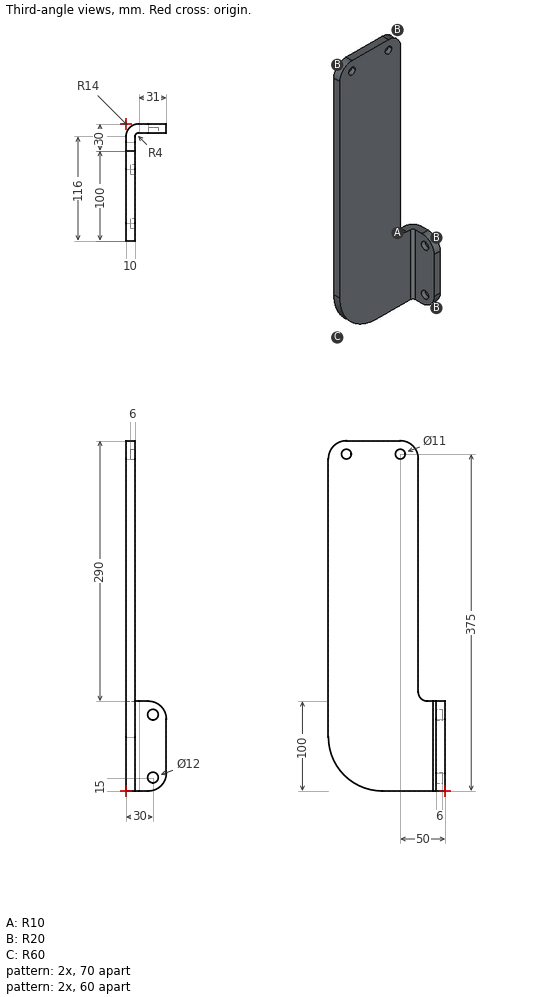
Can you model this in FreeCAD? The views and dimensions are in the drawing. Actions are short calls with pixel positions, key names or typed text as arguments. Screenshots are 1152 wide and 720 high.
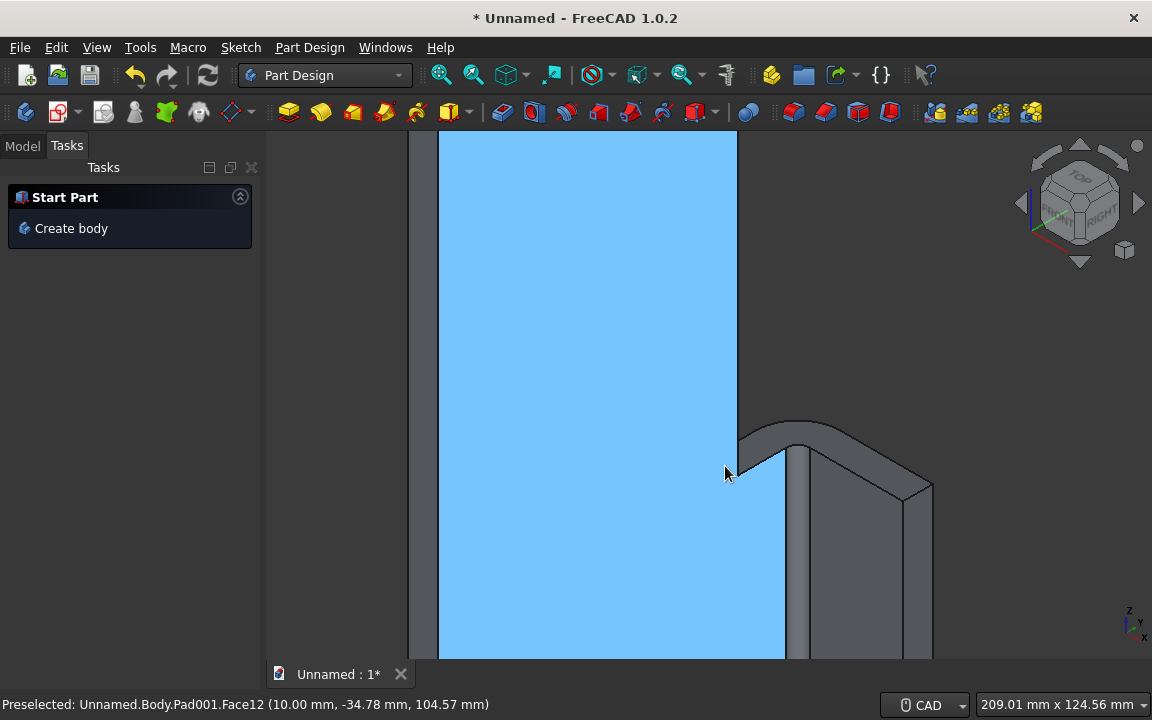
click(442, 76)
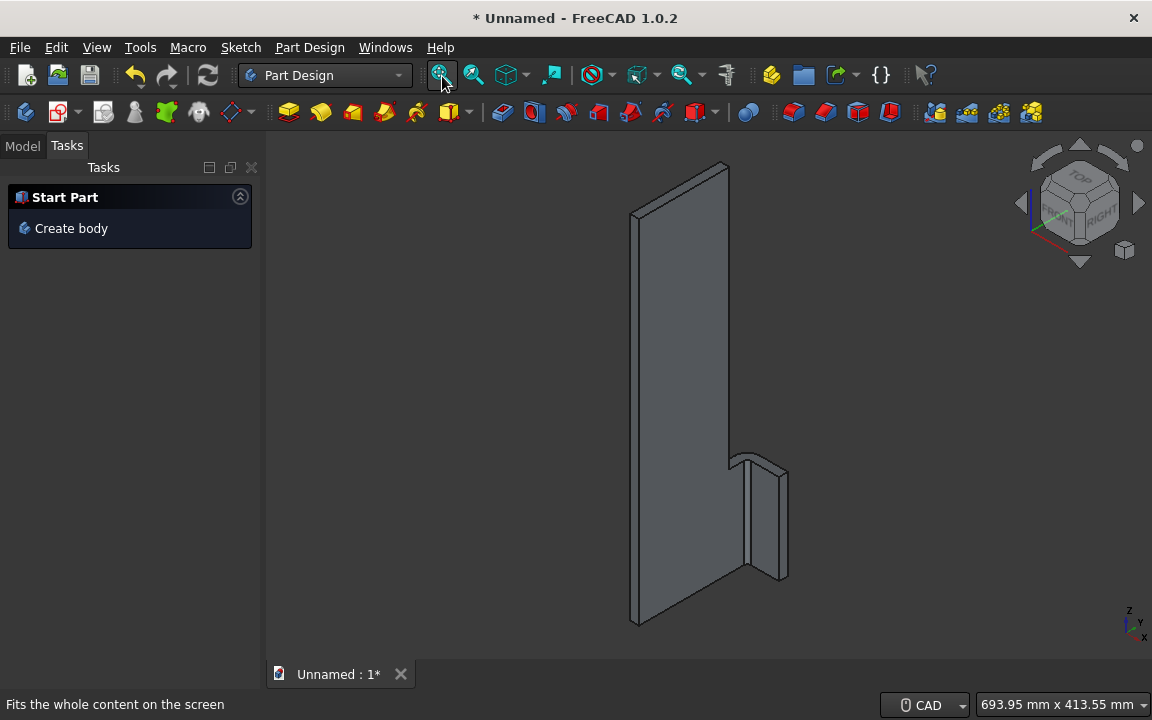
key(2)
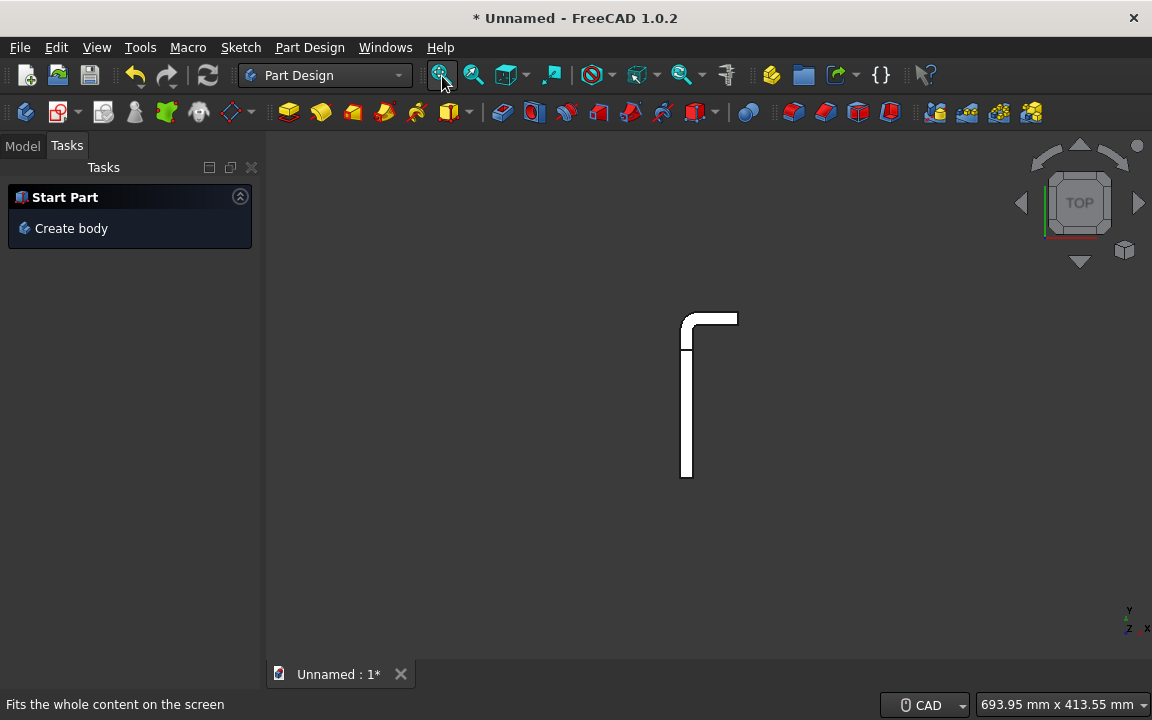
click(442, 76)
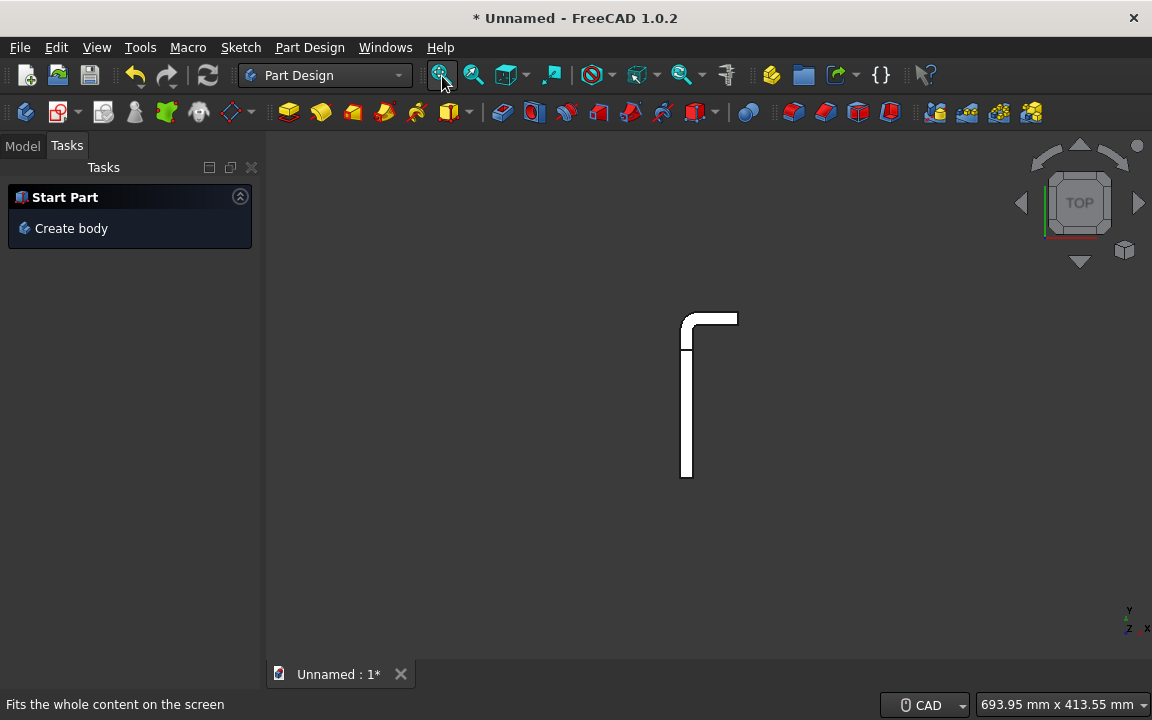
scroll(687, 349, up, 6)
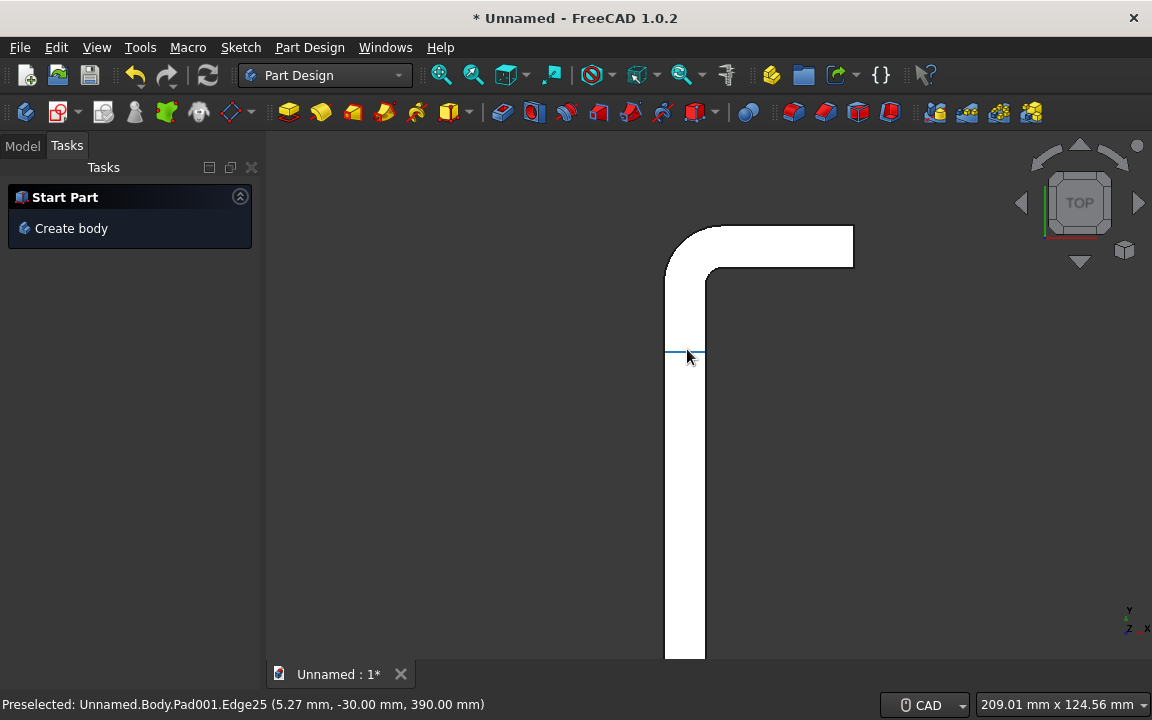
click(442, 76)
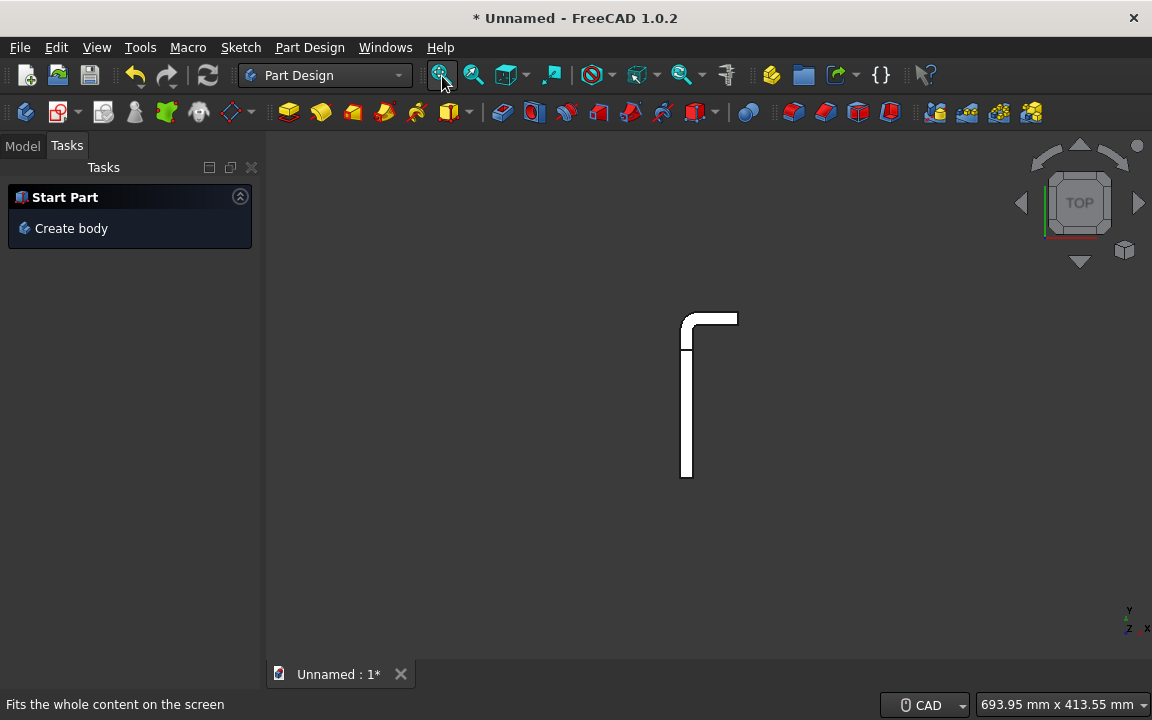
key(1)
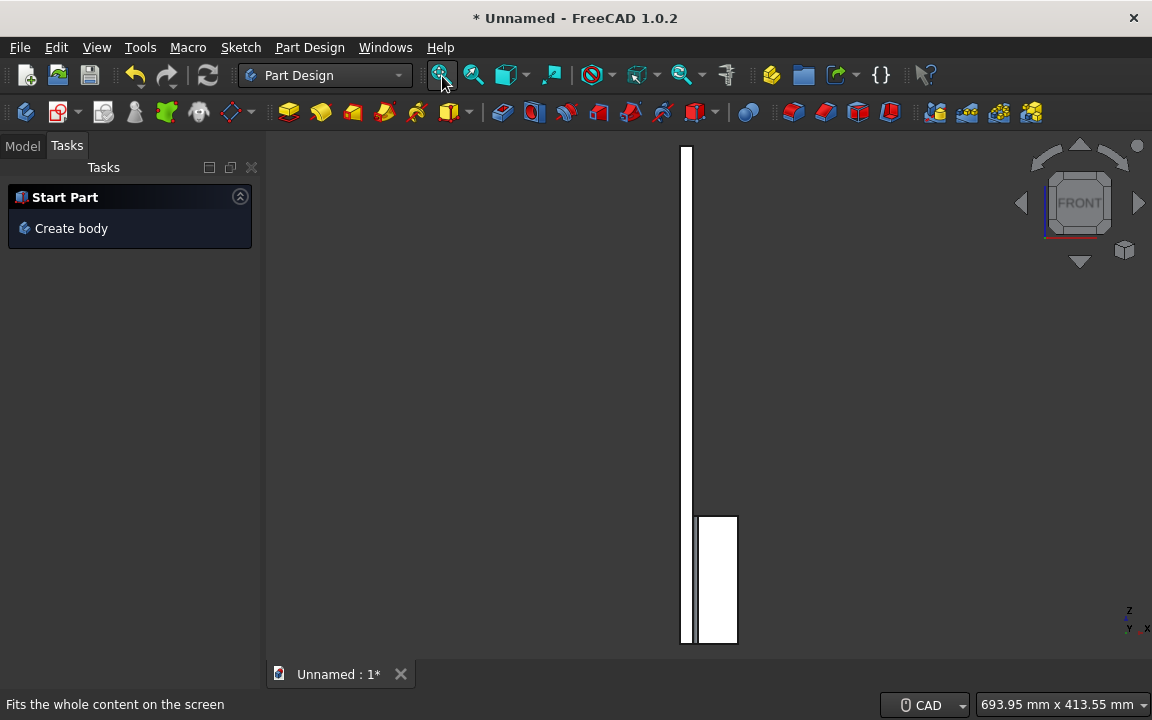
scroll(687, 515, up, 6)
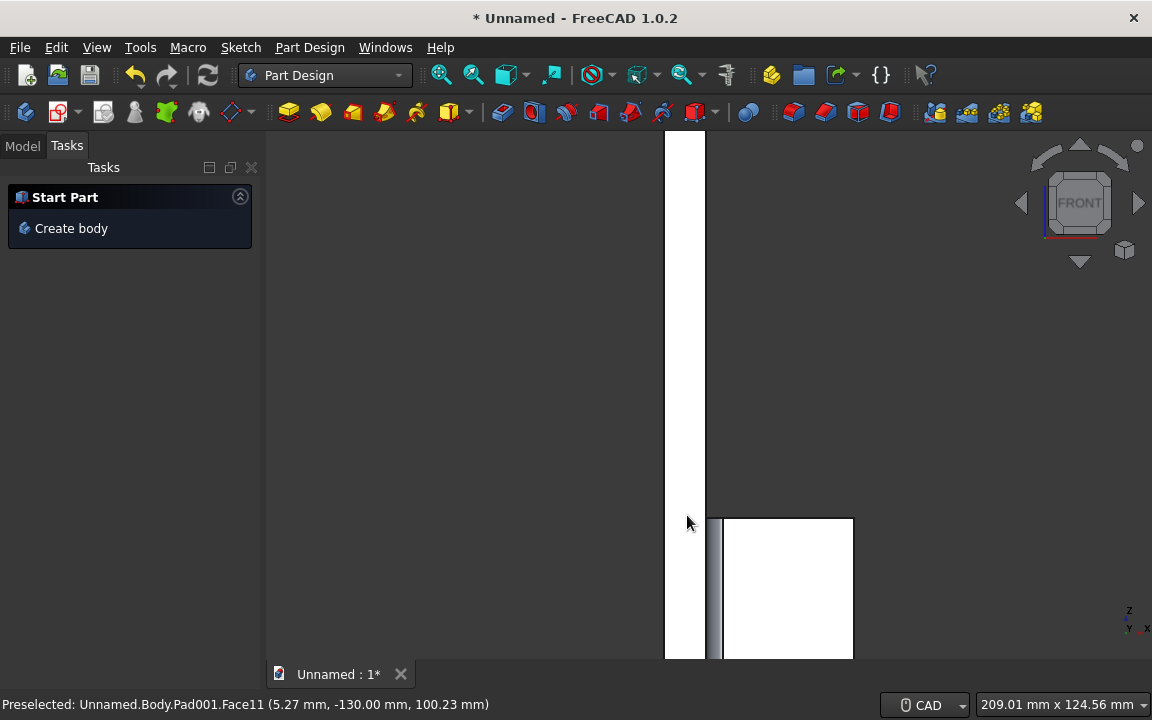
click(442, 76)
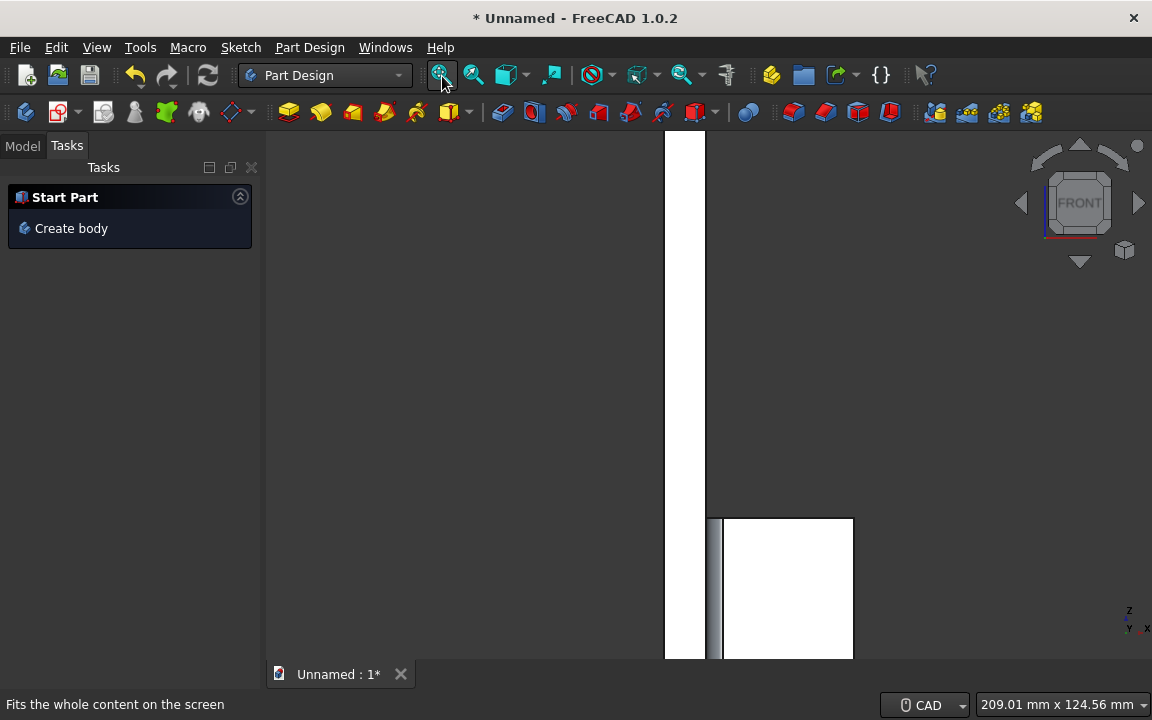
key(3)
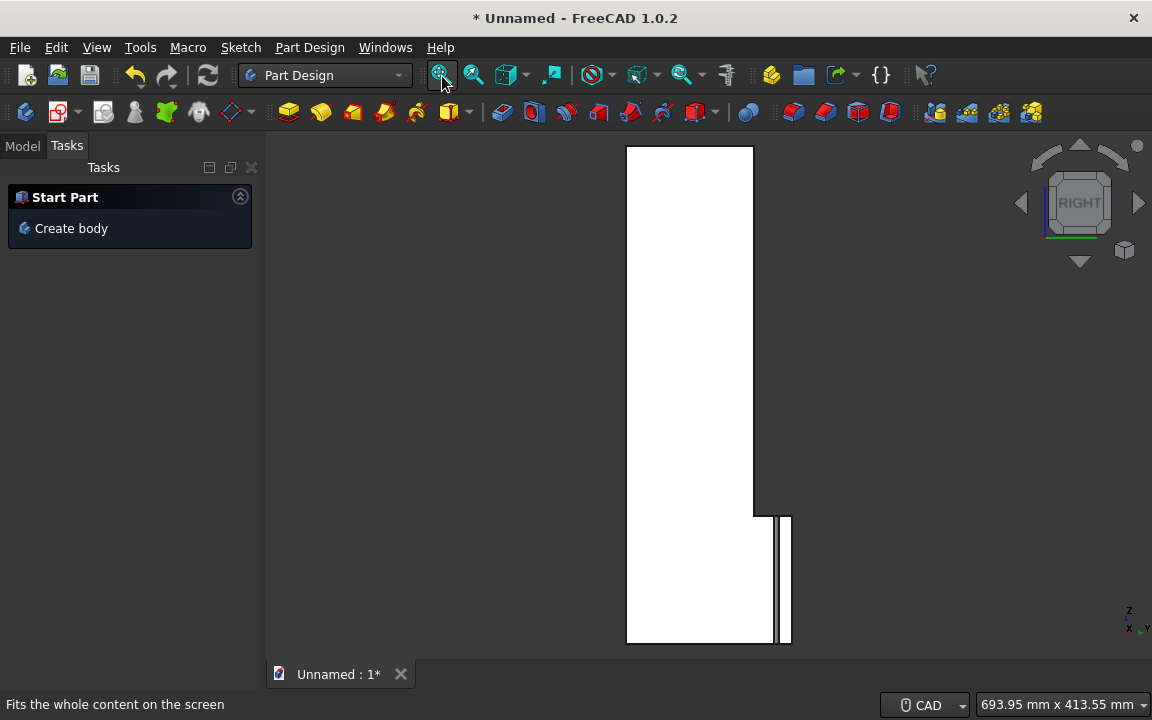
scroll(754, 515, up, 6)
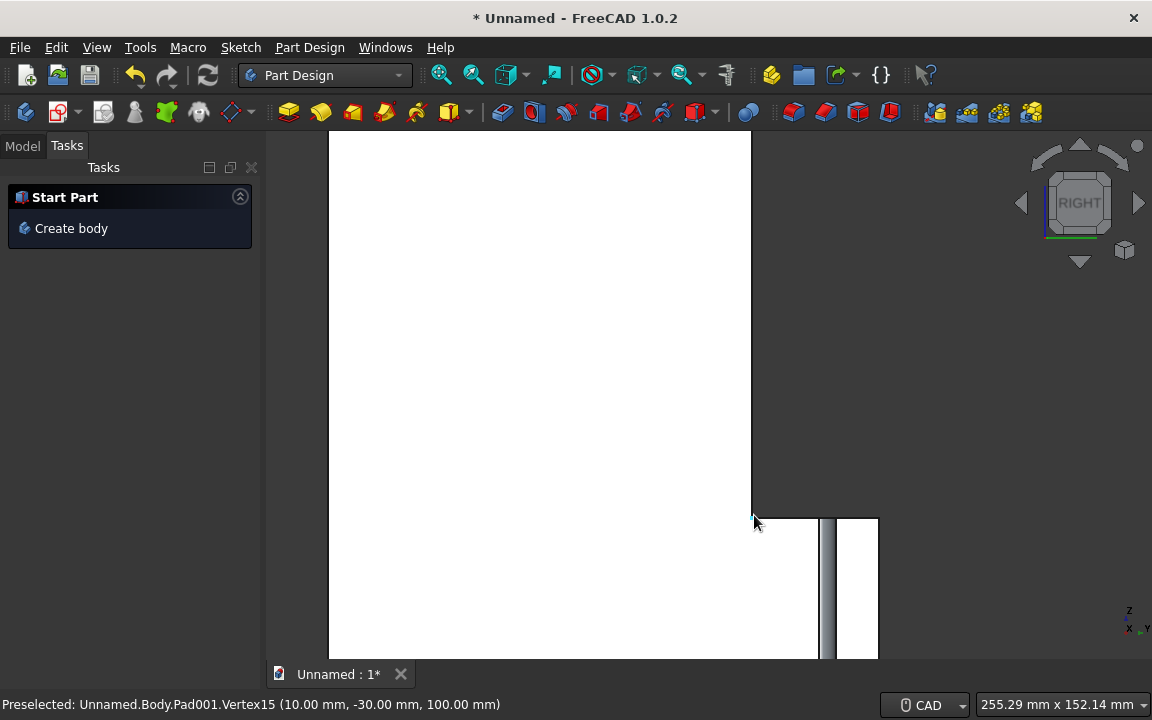
click(442, 76)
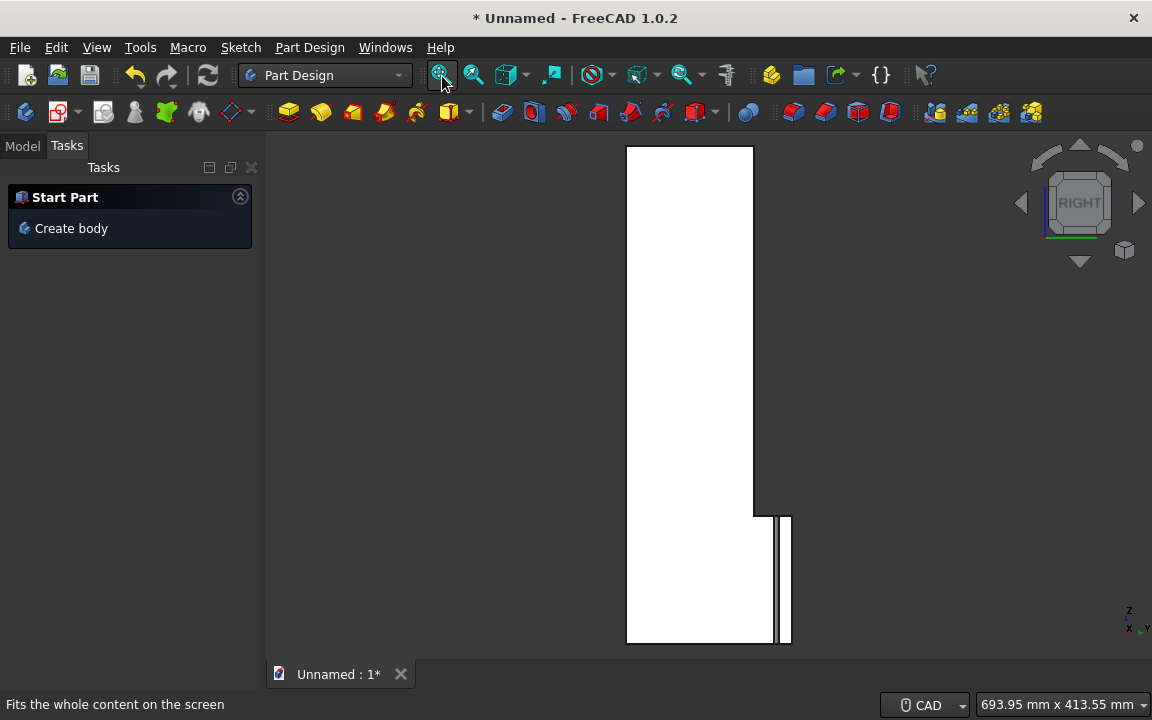
key(5)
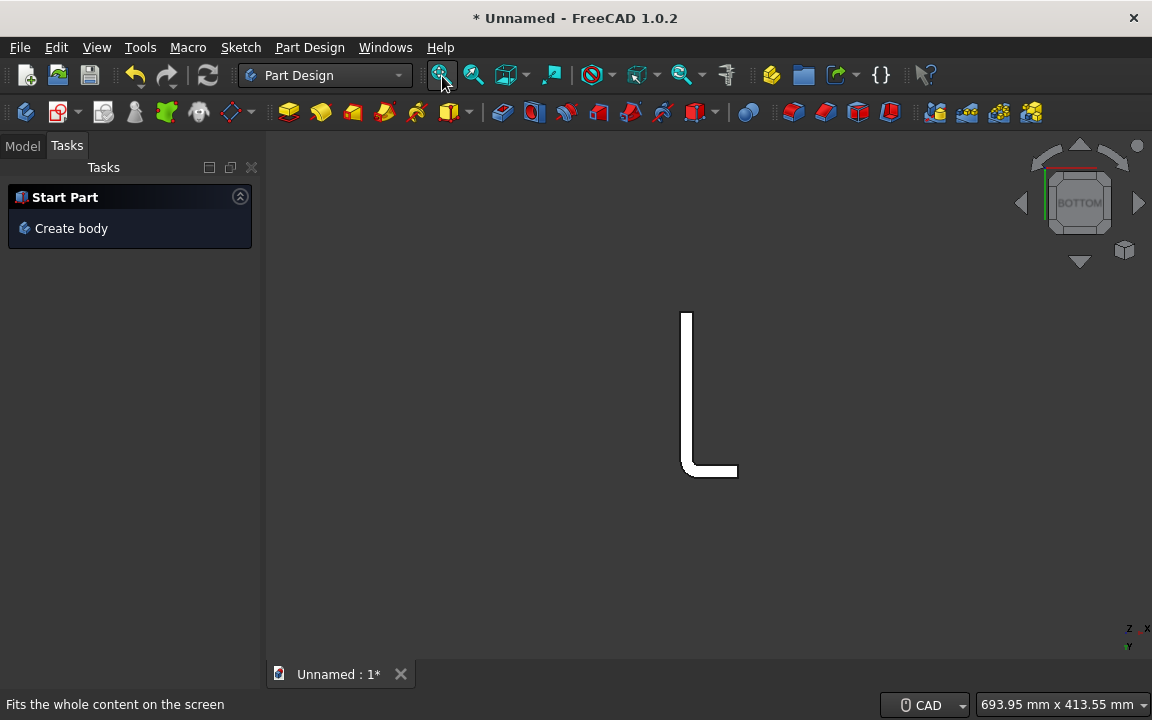
click(442, 76)